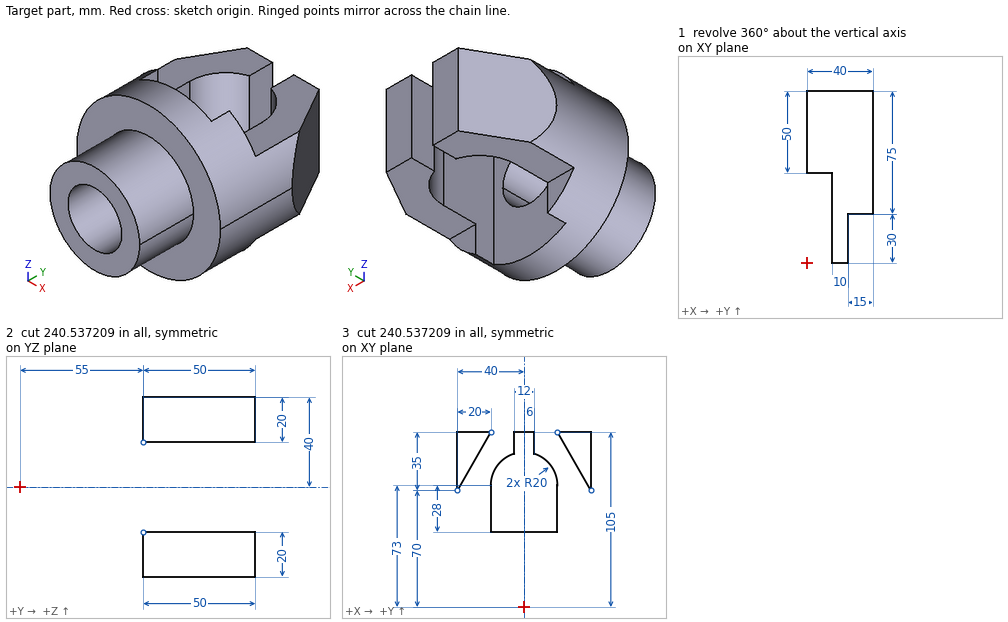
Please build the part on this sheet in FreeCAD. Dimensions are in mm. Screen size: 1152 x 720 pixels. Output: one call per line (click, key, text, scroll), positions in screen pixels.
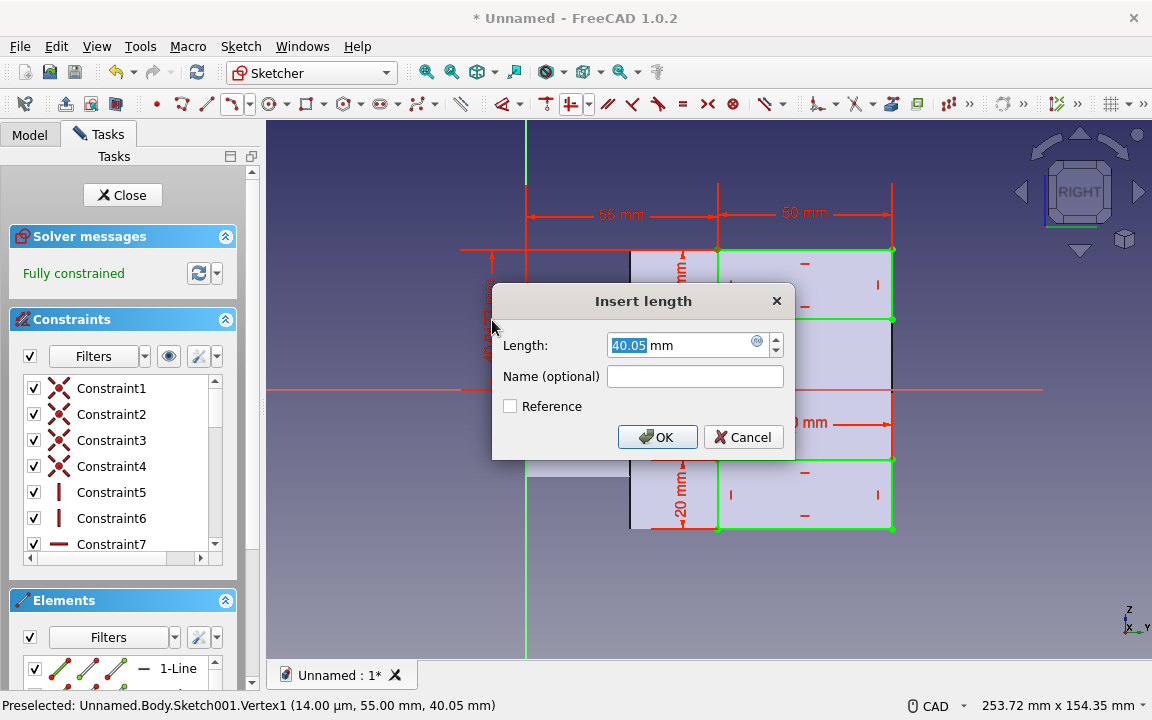
text(40)
key(Return)
key(Escape)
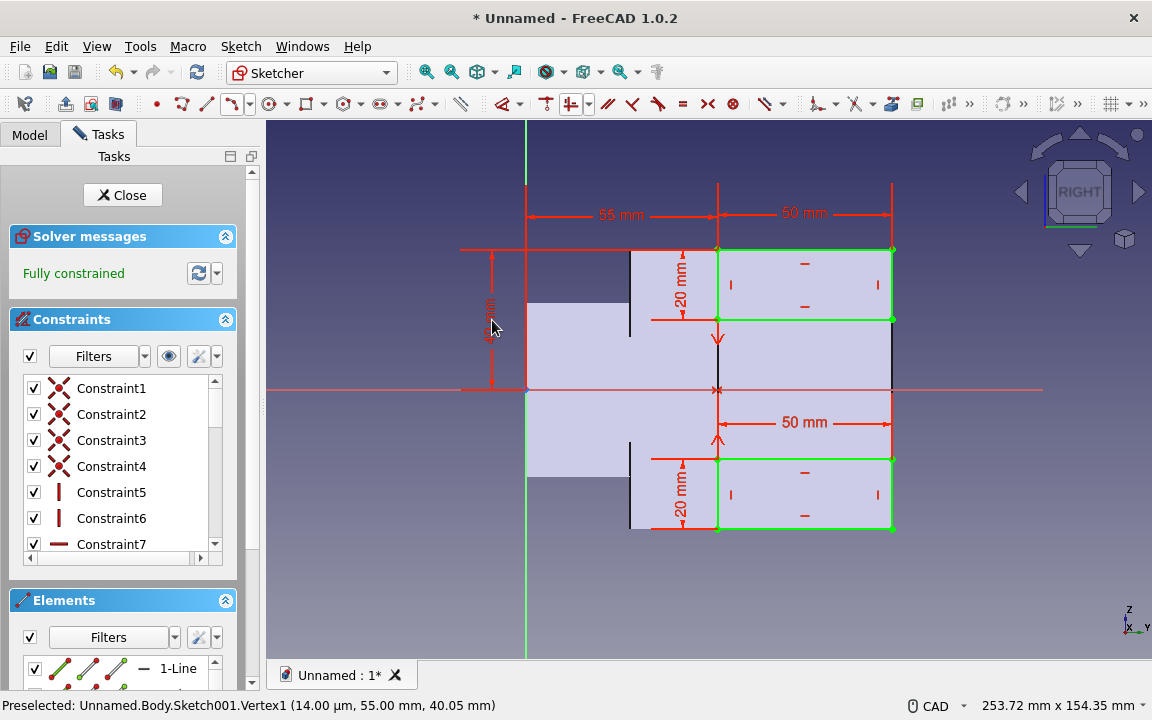
click(123, 195)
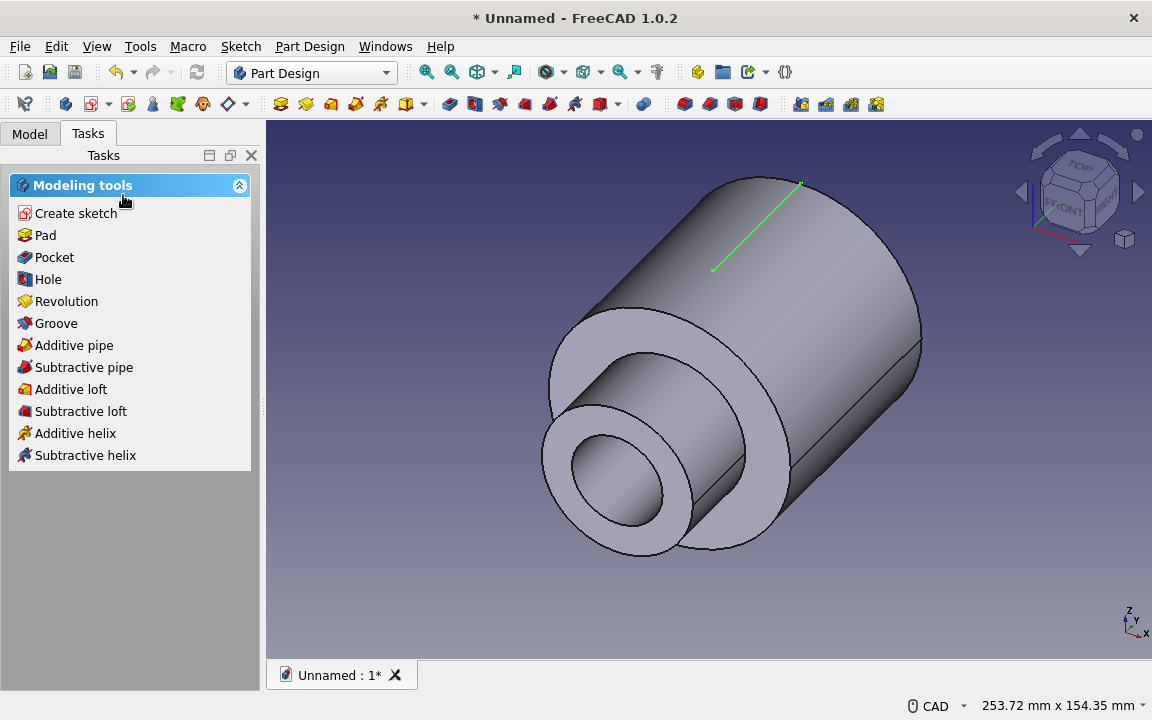
click(450, 104)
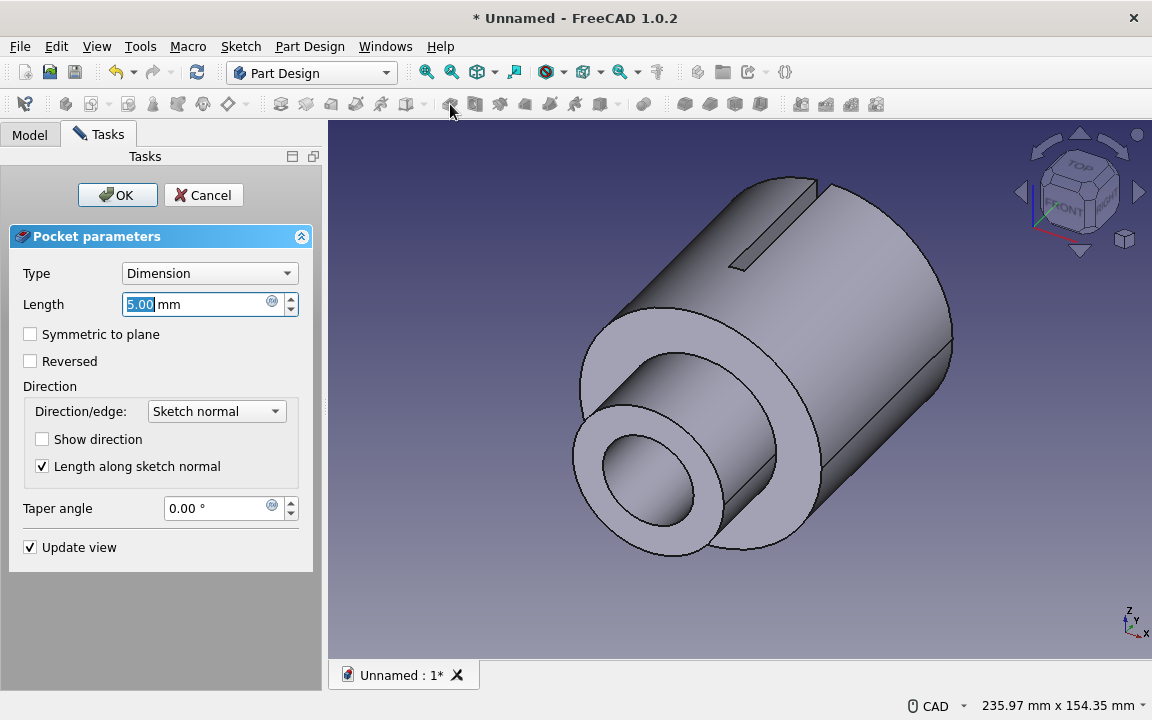
text(240.537209)
key(Tab)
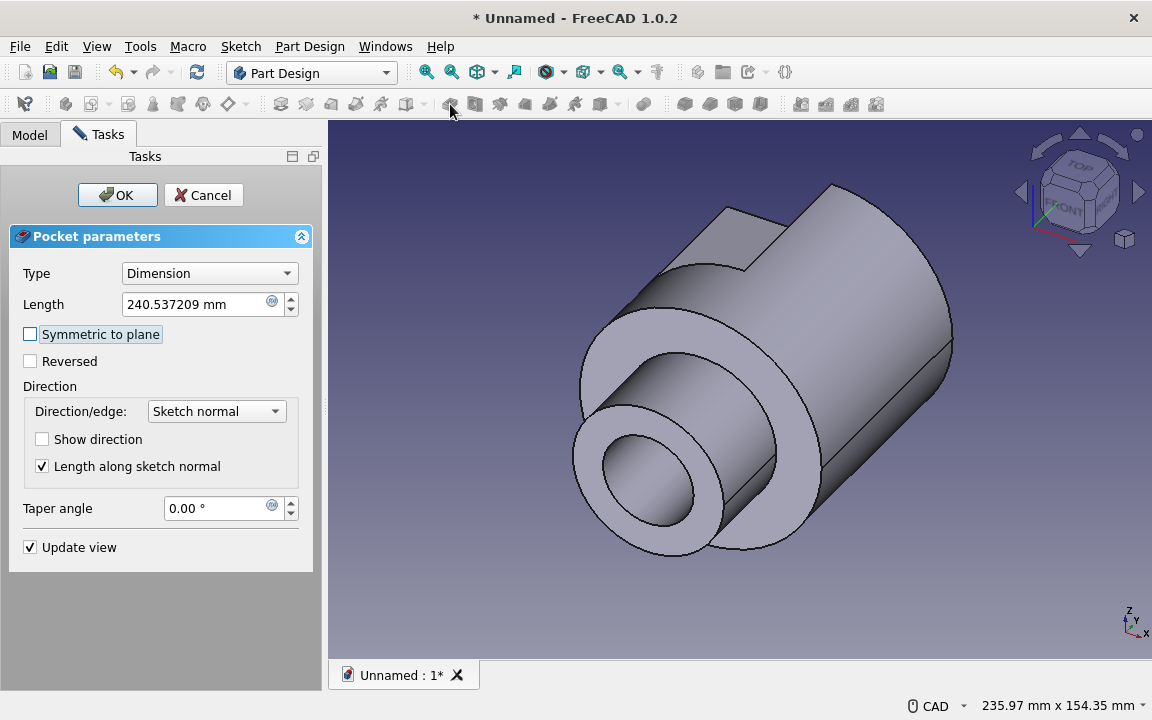
click(31, 334)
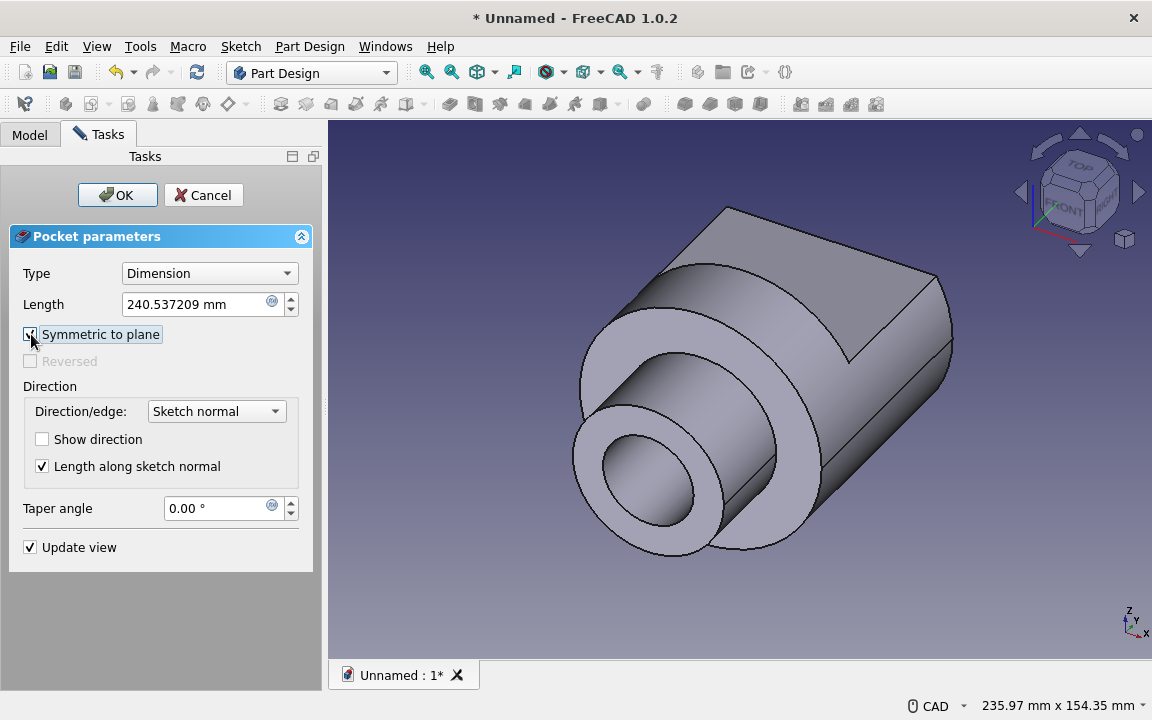
click(118, 195)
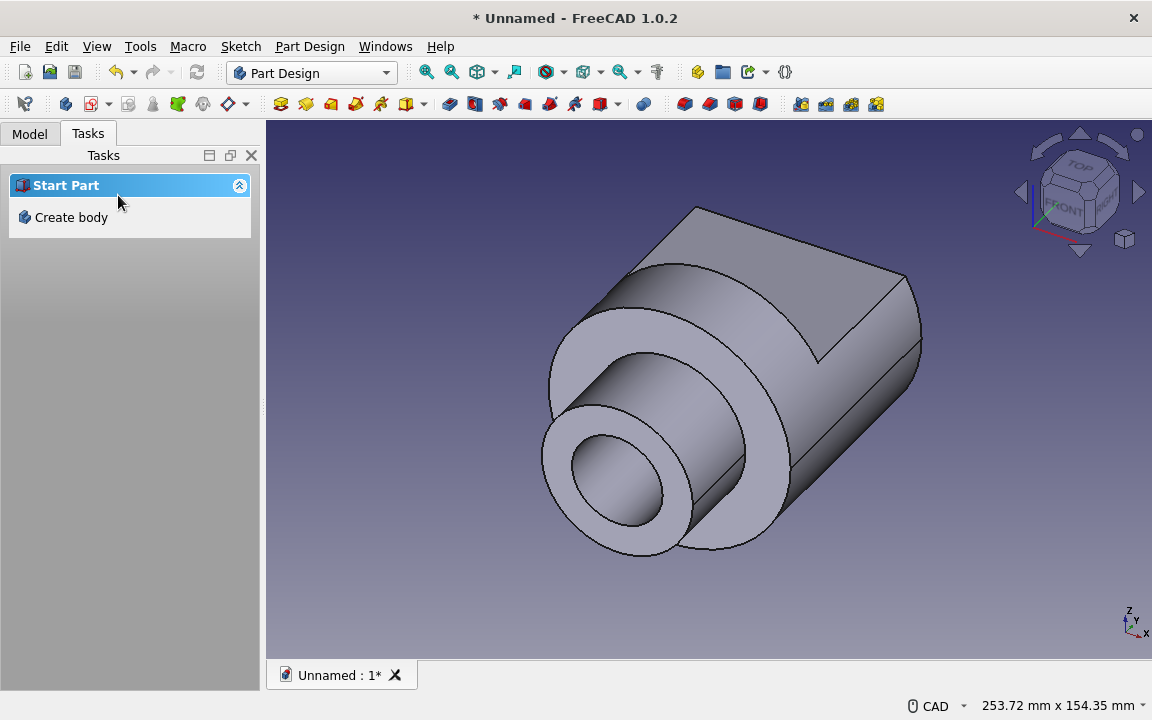
click(90, 104)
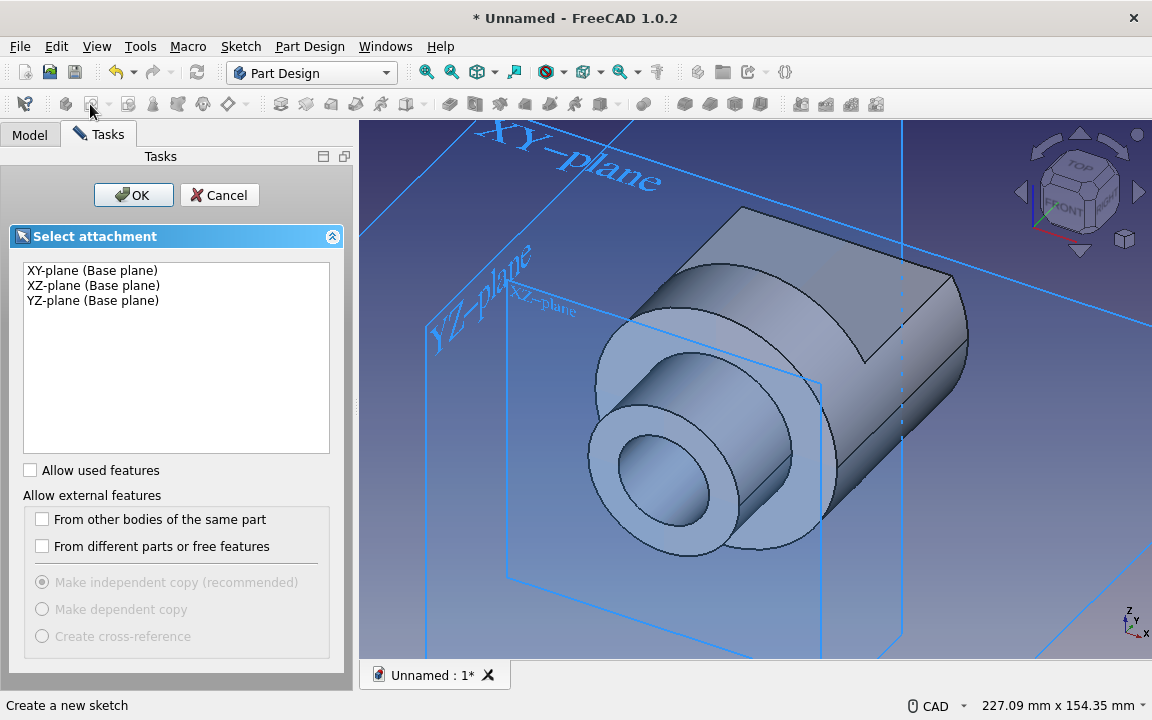
click(84, 270)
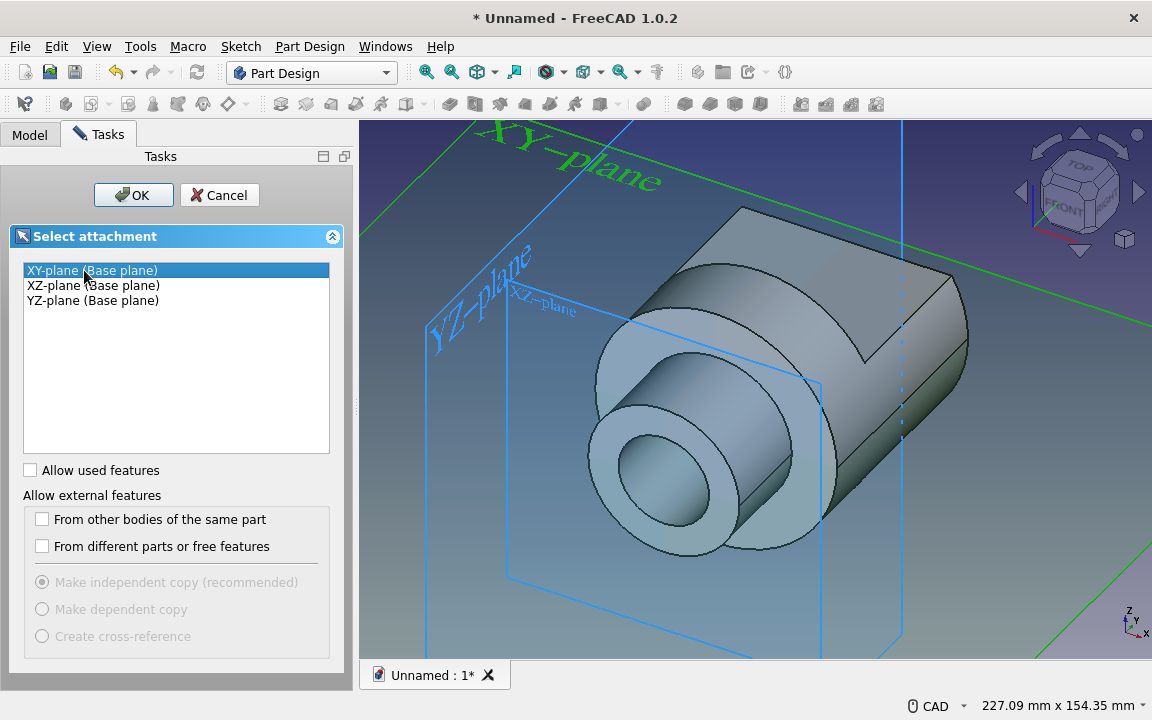
click(134, 195)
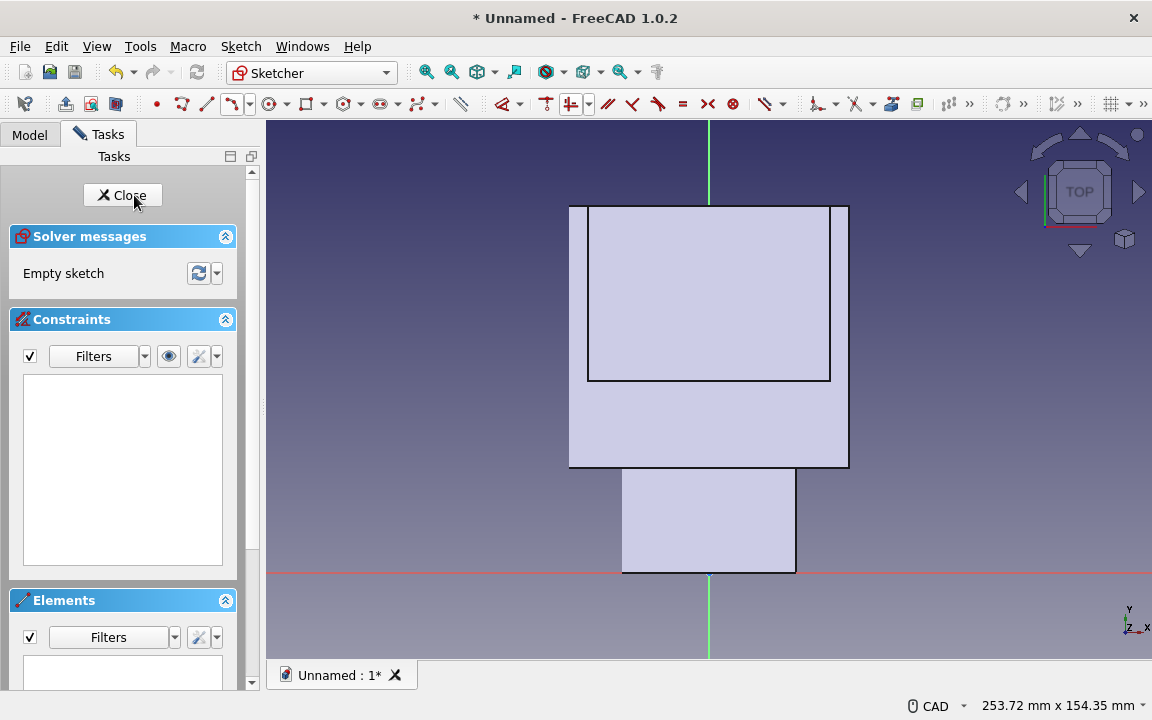
click(116, 104)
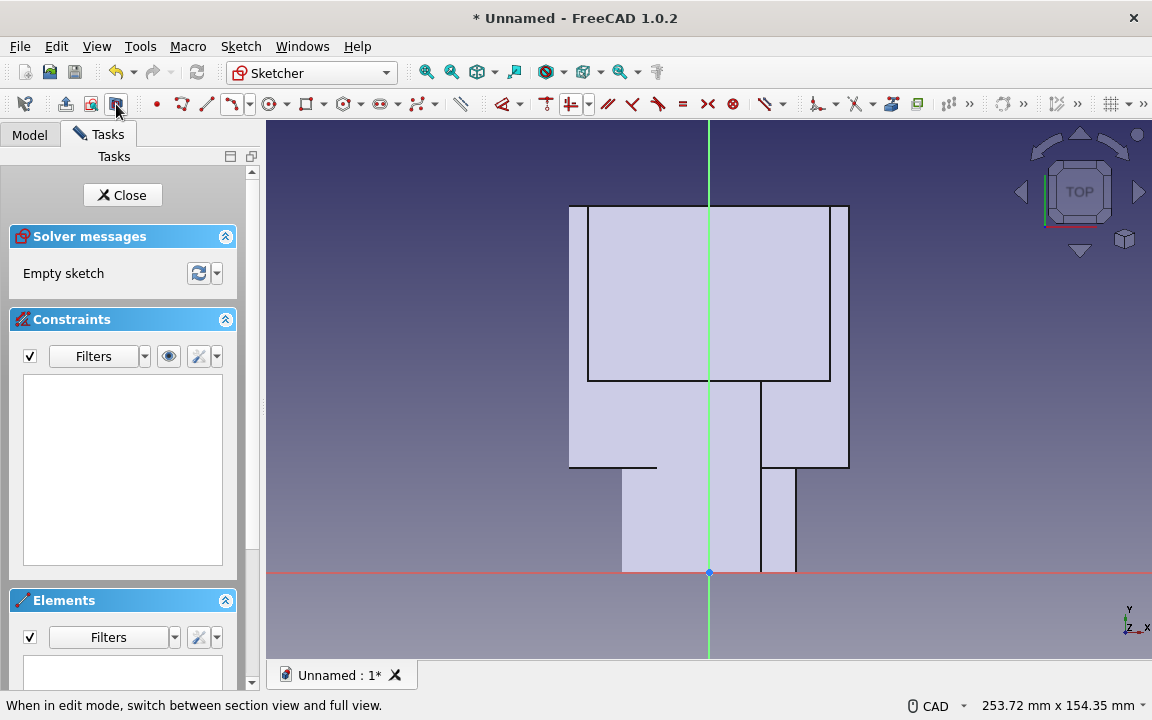
click(182, 104)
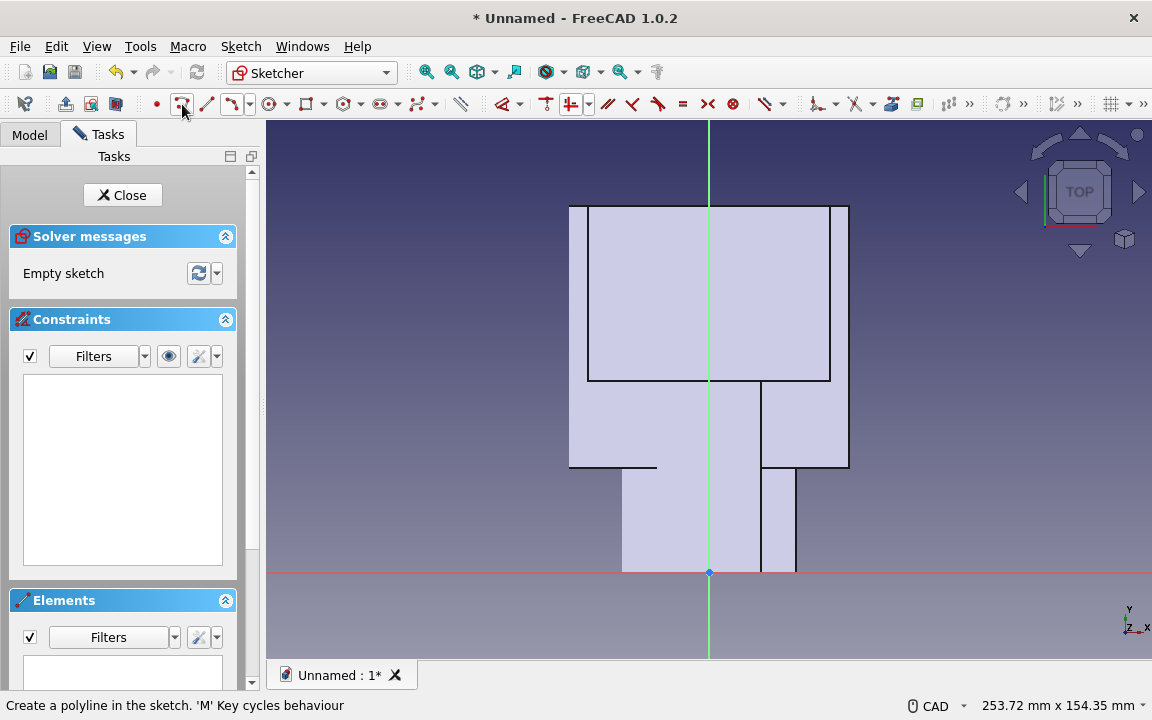
click(569, 328)
click(639, 206)
click(569, 206)
click(569, 329)